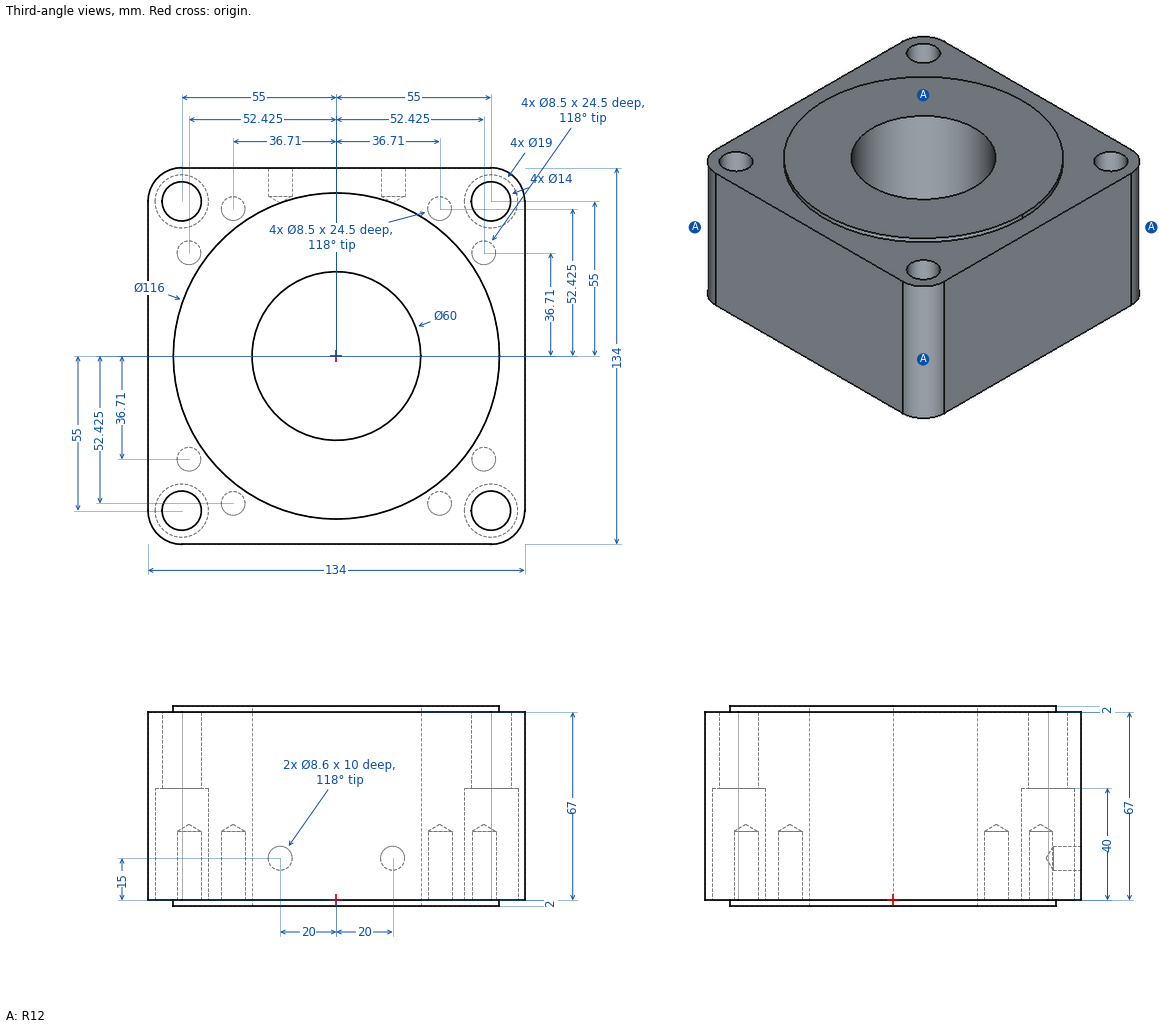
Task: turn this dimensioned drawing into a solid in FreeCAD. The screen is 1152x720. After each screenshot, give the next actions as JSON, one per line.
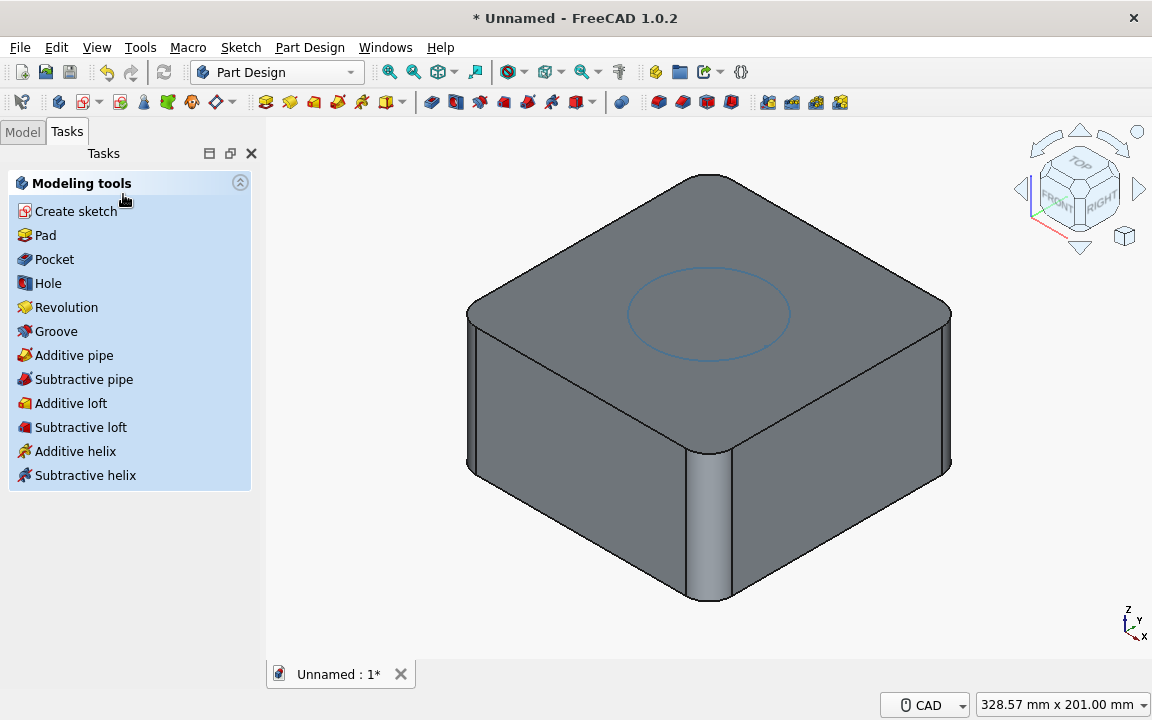
{"action": "left_click", "coordinate": [432, 102]}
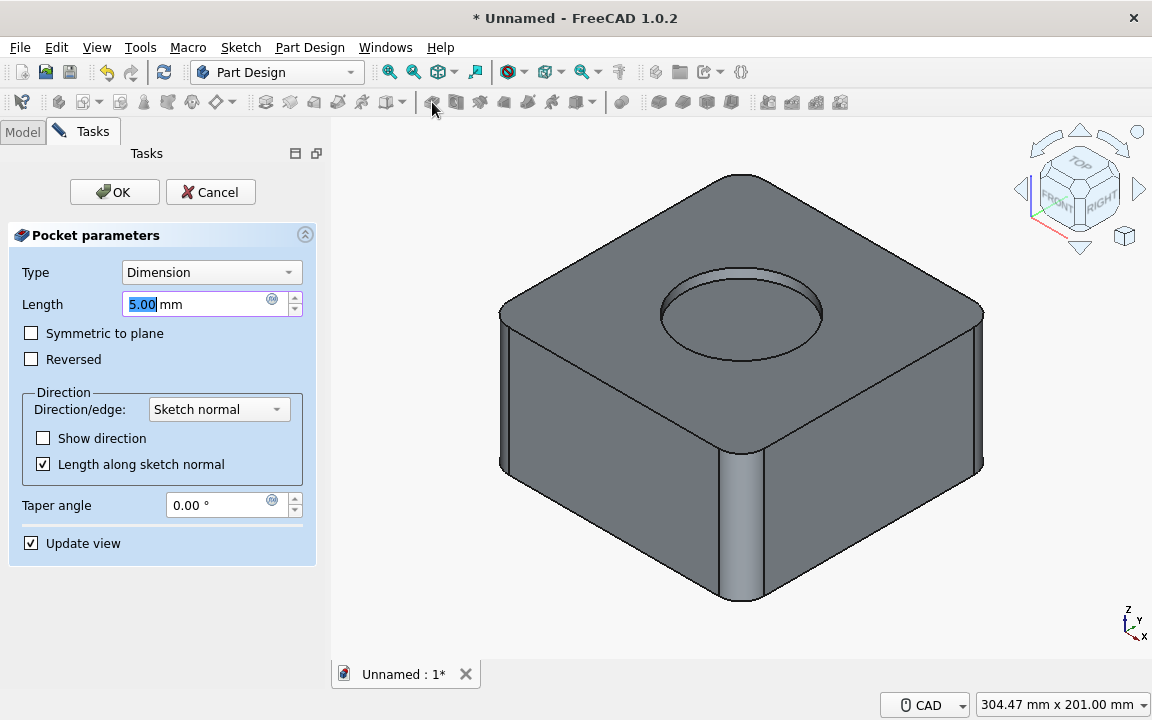
{"action": "type", "text": "67"}
{"action": "key", "text": "Tab"}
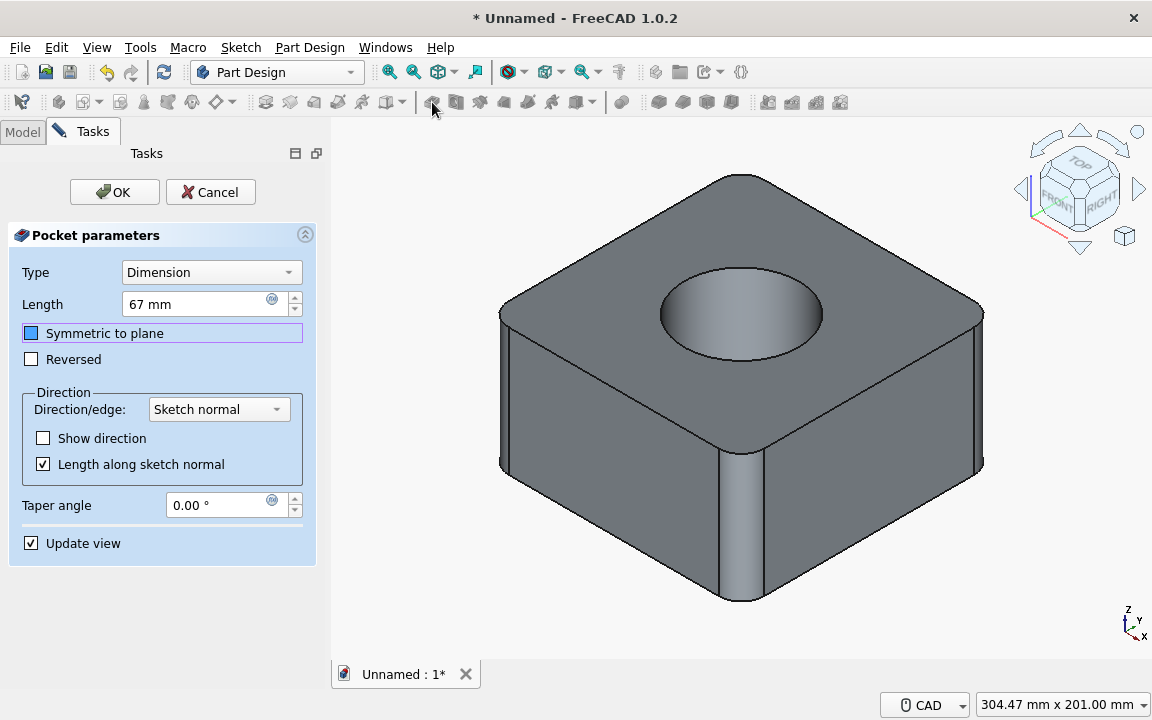
{"action": "left_click", "coordinate": [115, 192]}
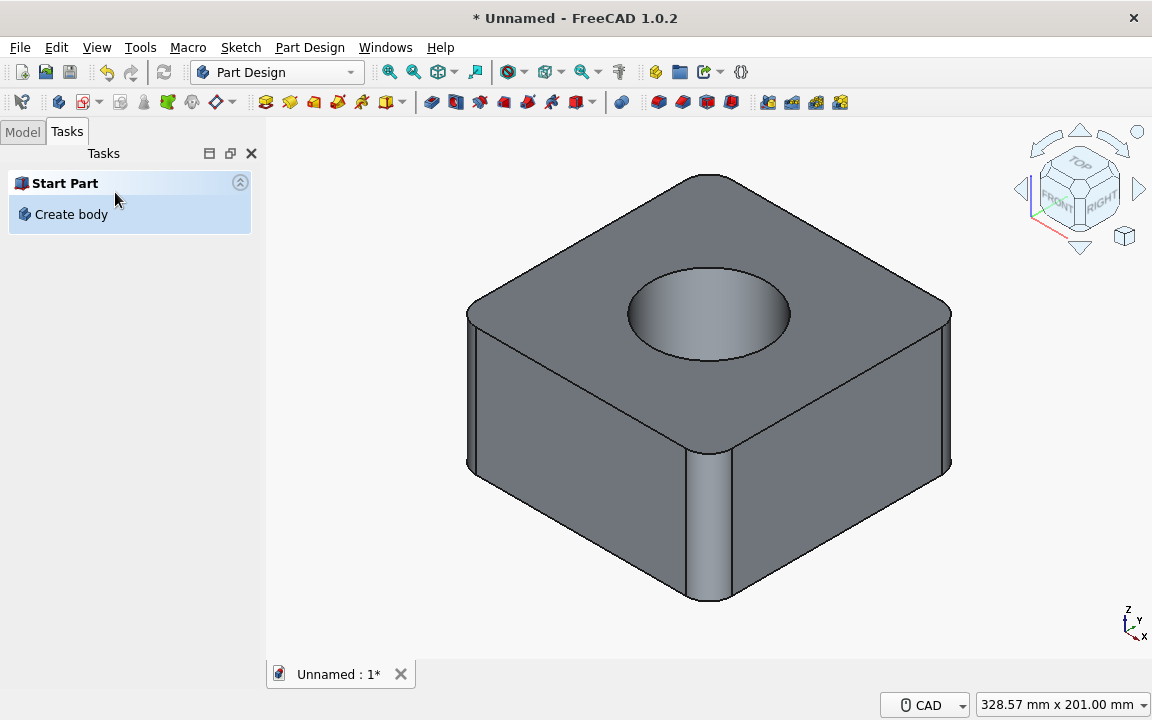
{"action": "left_click", "coordinate": [23, 131]}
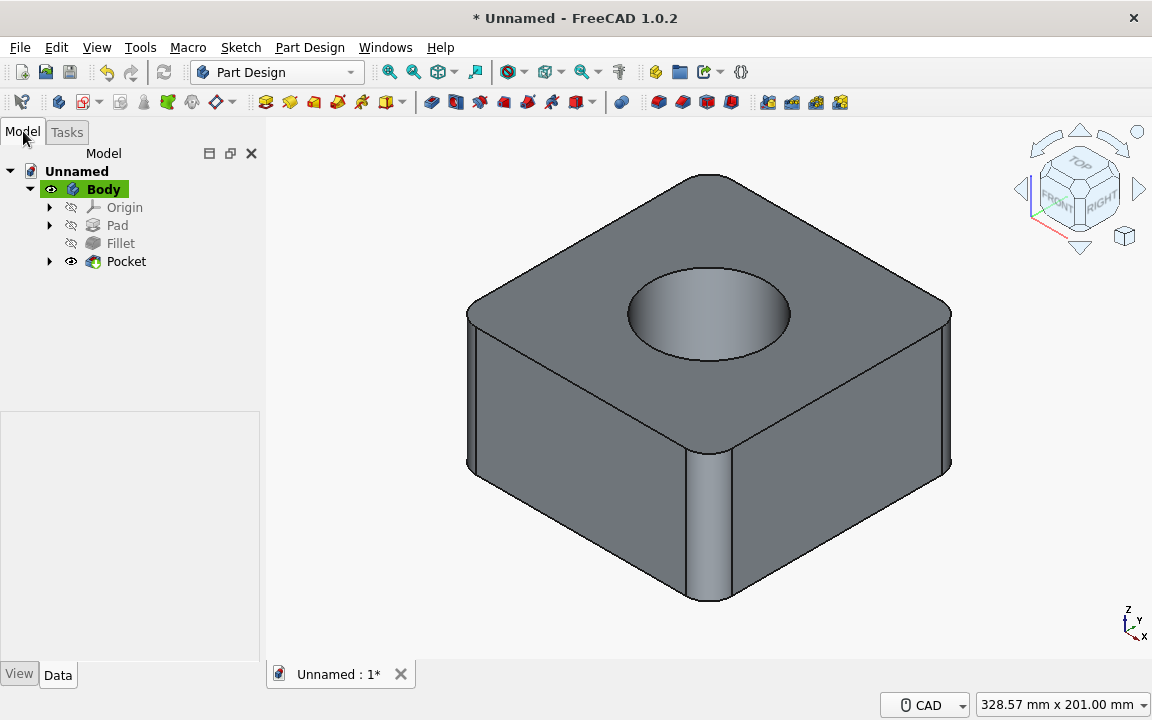
{"action": "left_click", "coordinate": [50, 207]}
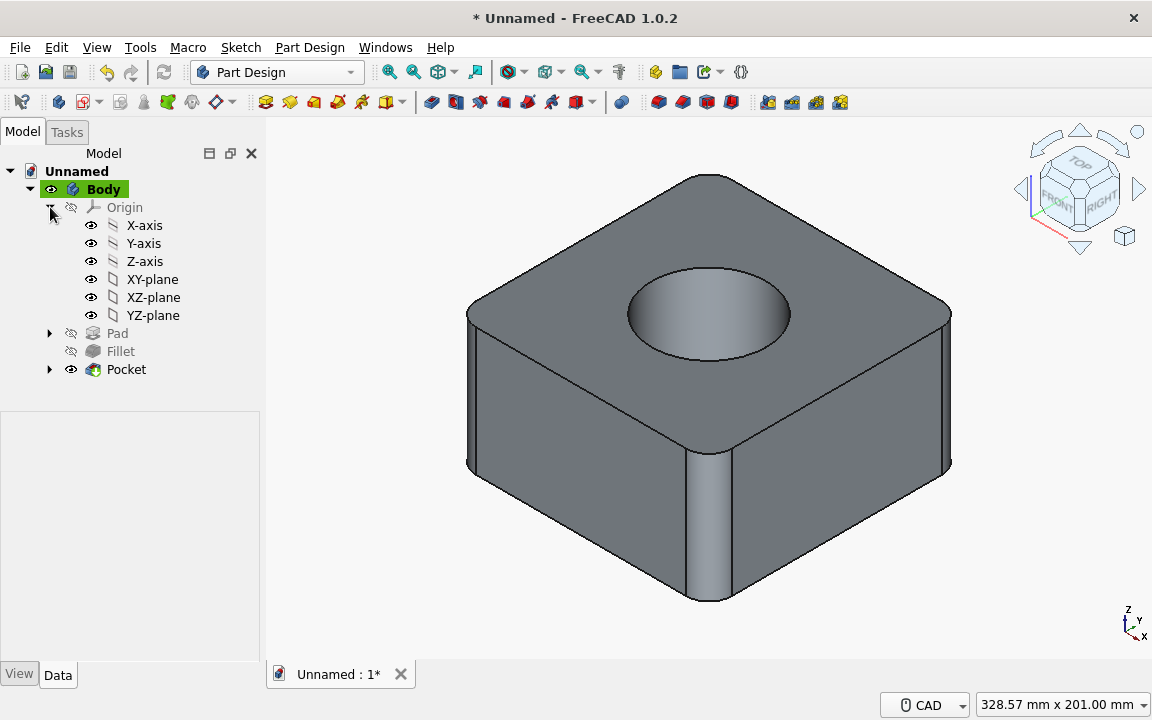
{"action": "left_click", "coordinate": [136, 279]}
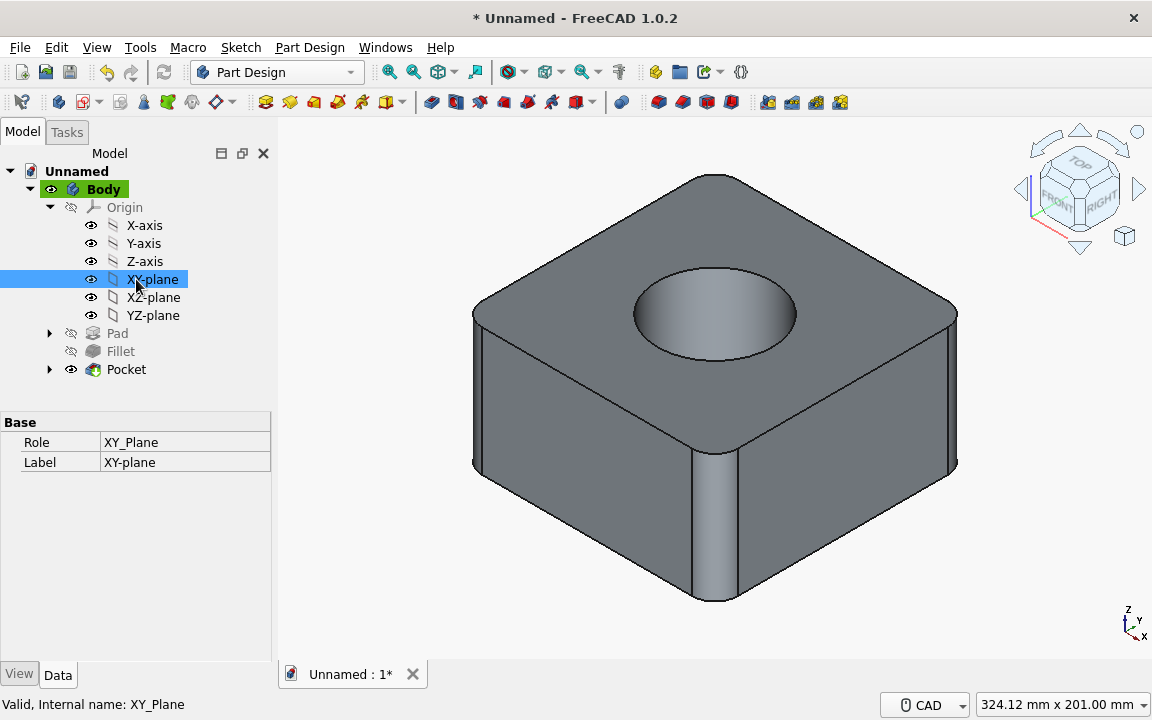
{"action": "left_click", "coordinate": [216, 102]}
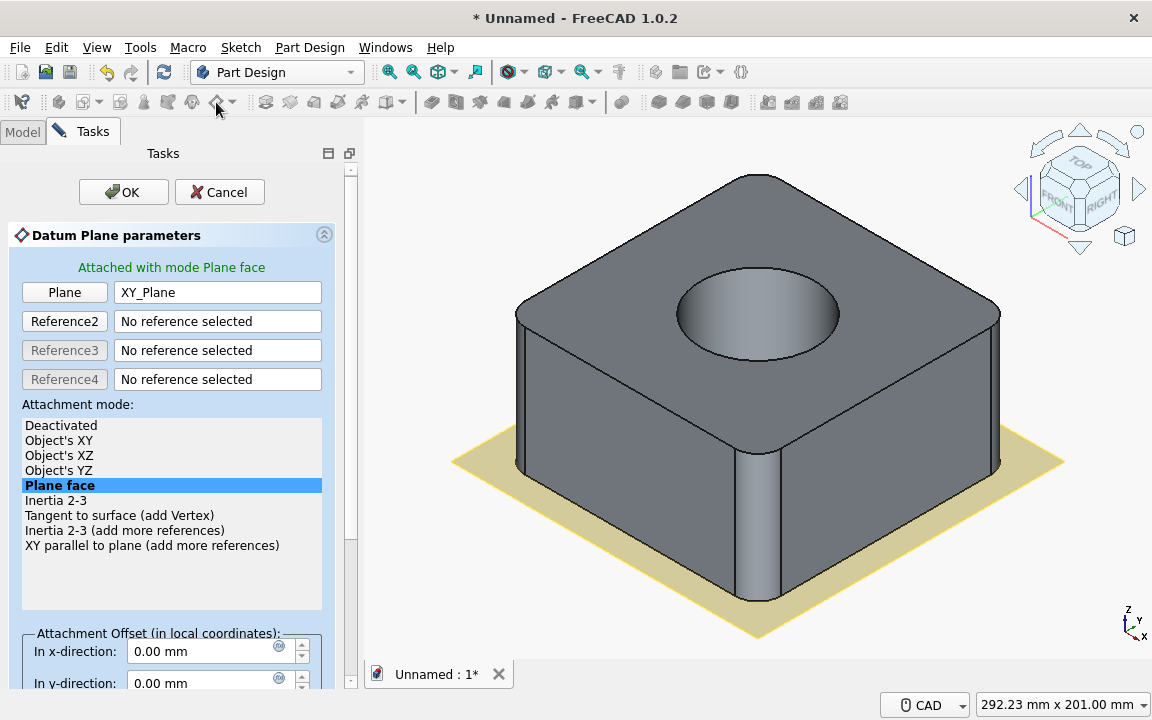
{"action": "scroll", "coordinate": [351, 426], "scroll_direction": "down", "scroll_amount": 2}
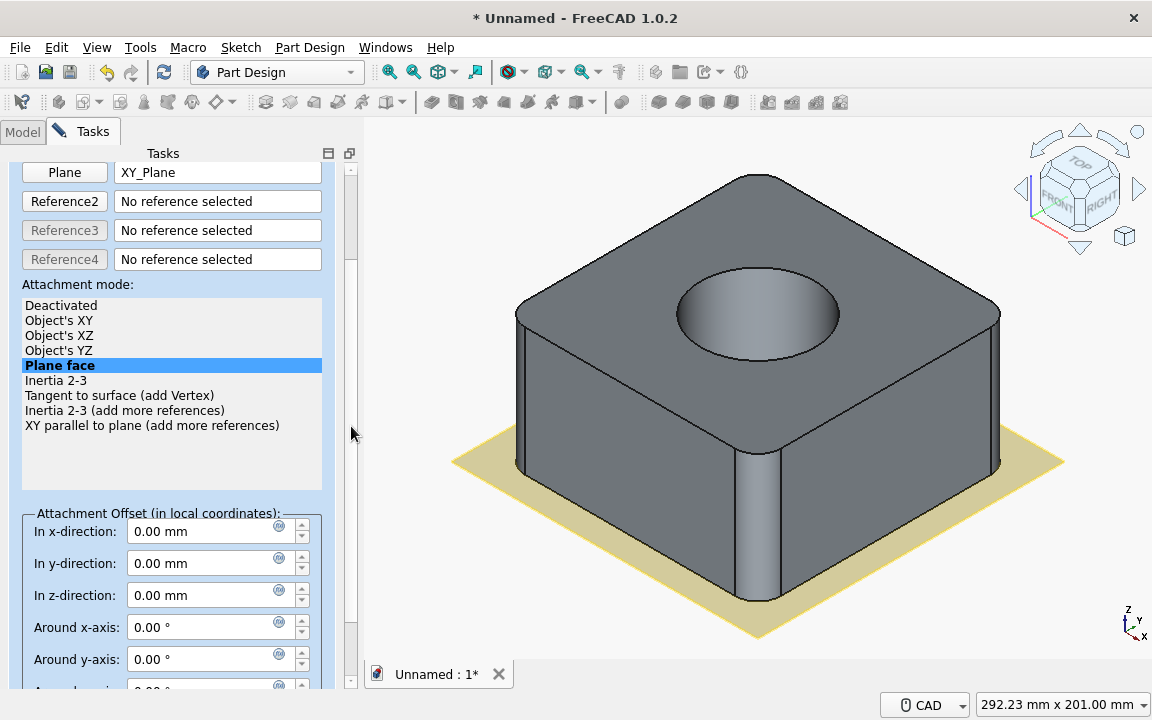
{"action": "triple_click", "coordinate": [210, 595]}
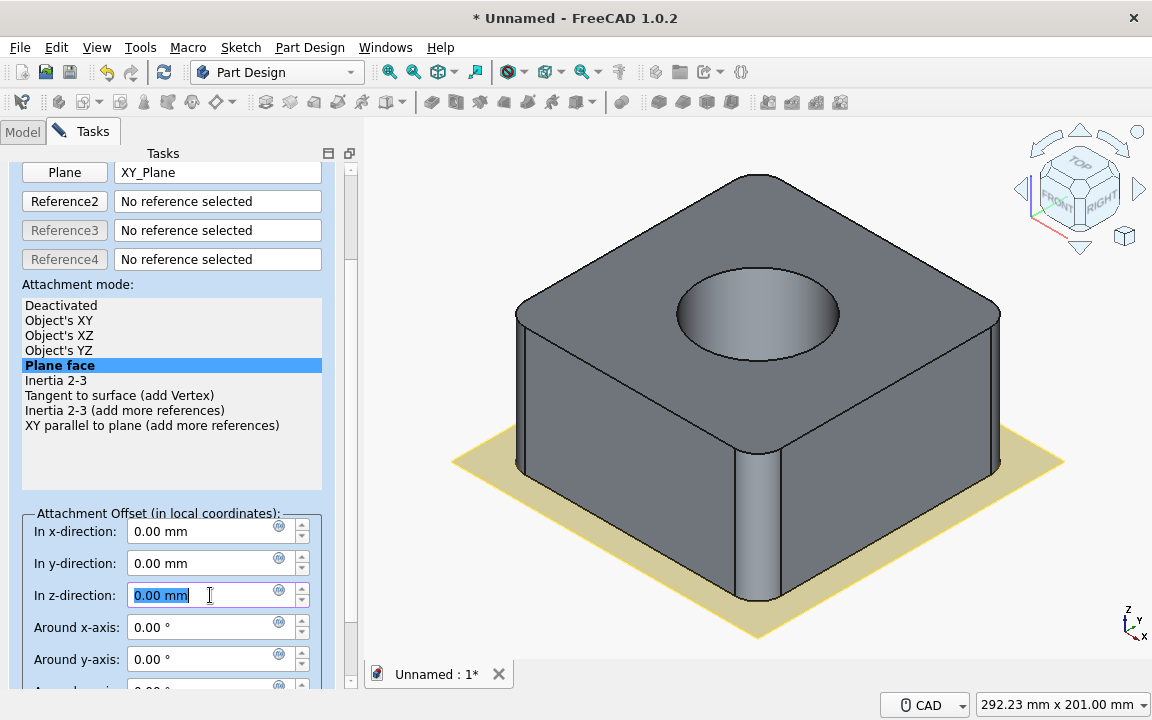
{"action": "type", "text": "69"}
{"action": "key", "text": "Tab"}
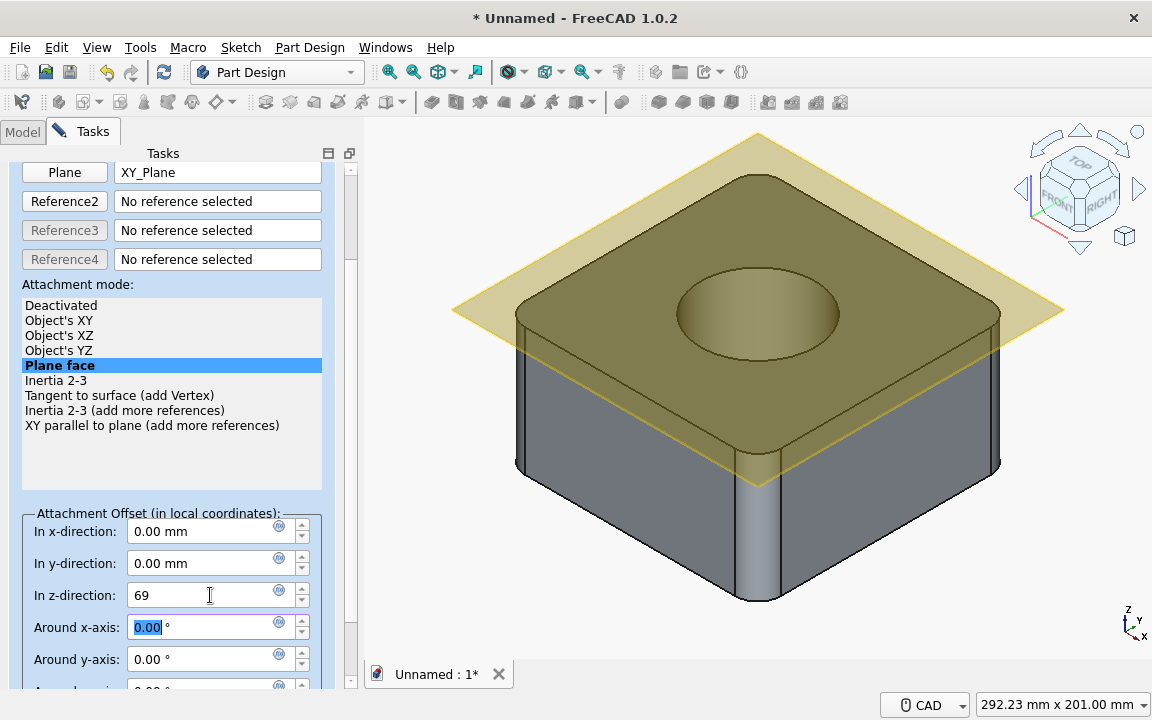
{"action": "scroll", "coordinate": [351, 426], "scroll_direction": "up", "scroll_amount": 3}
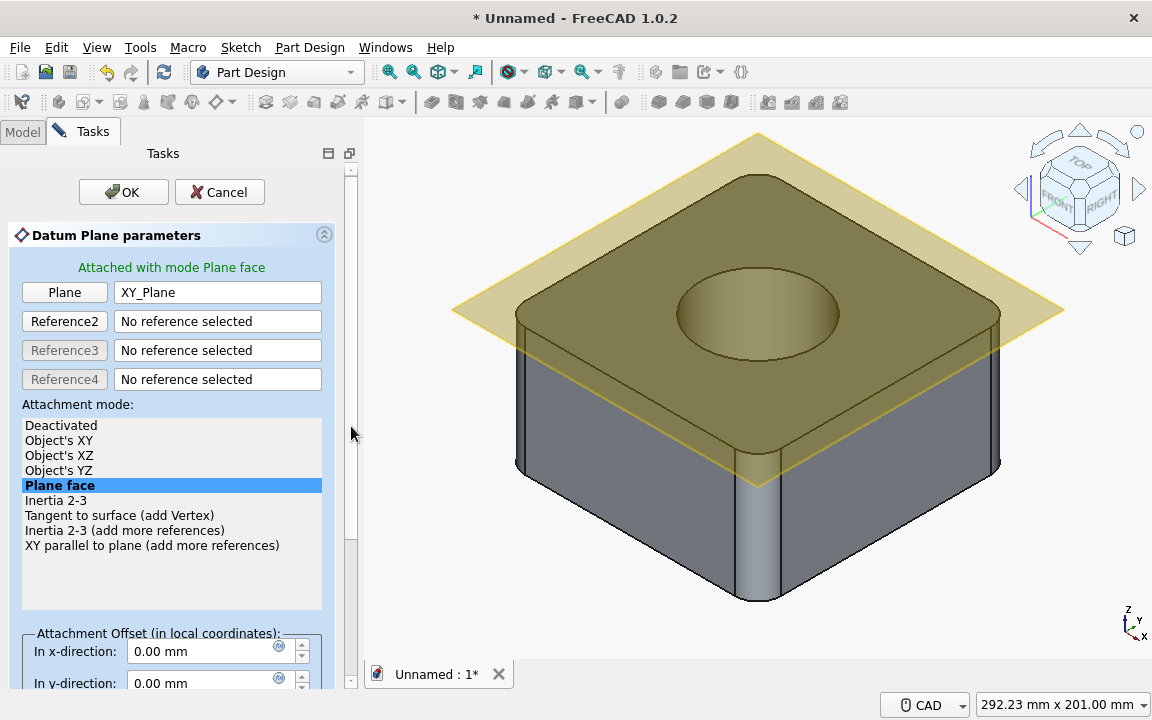
{"action": "left_click", "coordinate": [124, 192]}